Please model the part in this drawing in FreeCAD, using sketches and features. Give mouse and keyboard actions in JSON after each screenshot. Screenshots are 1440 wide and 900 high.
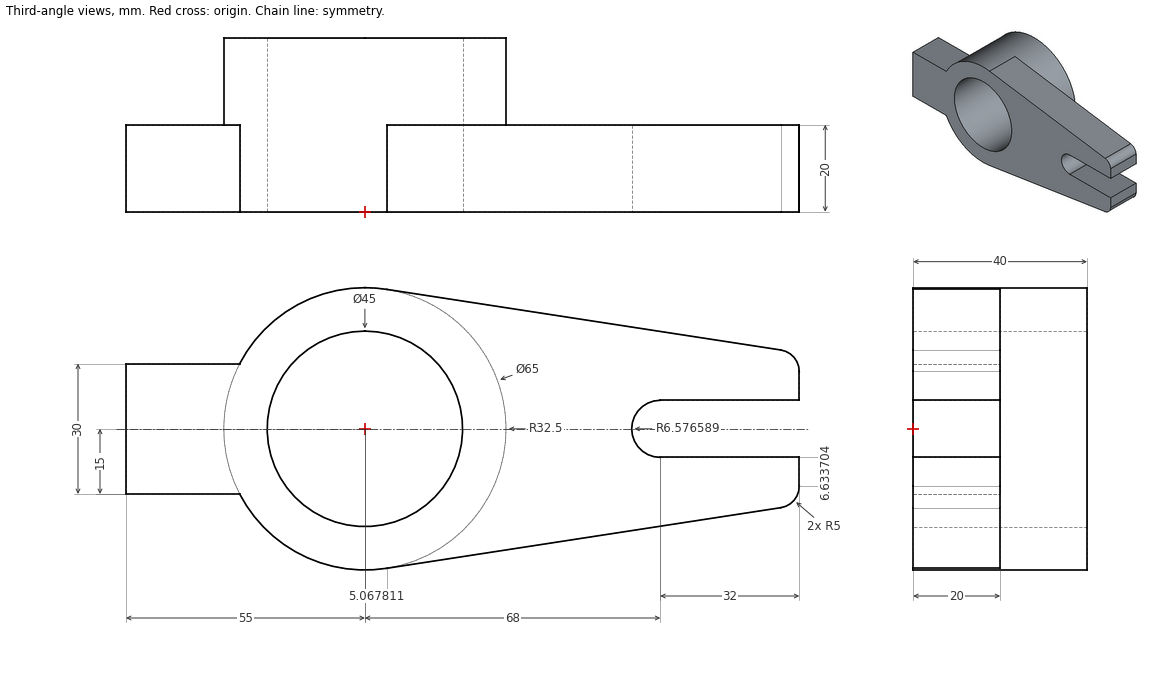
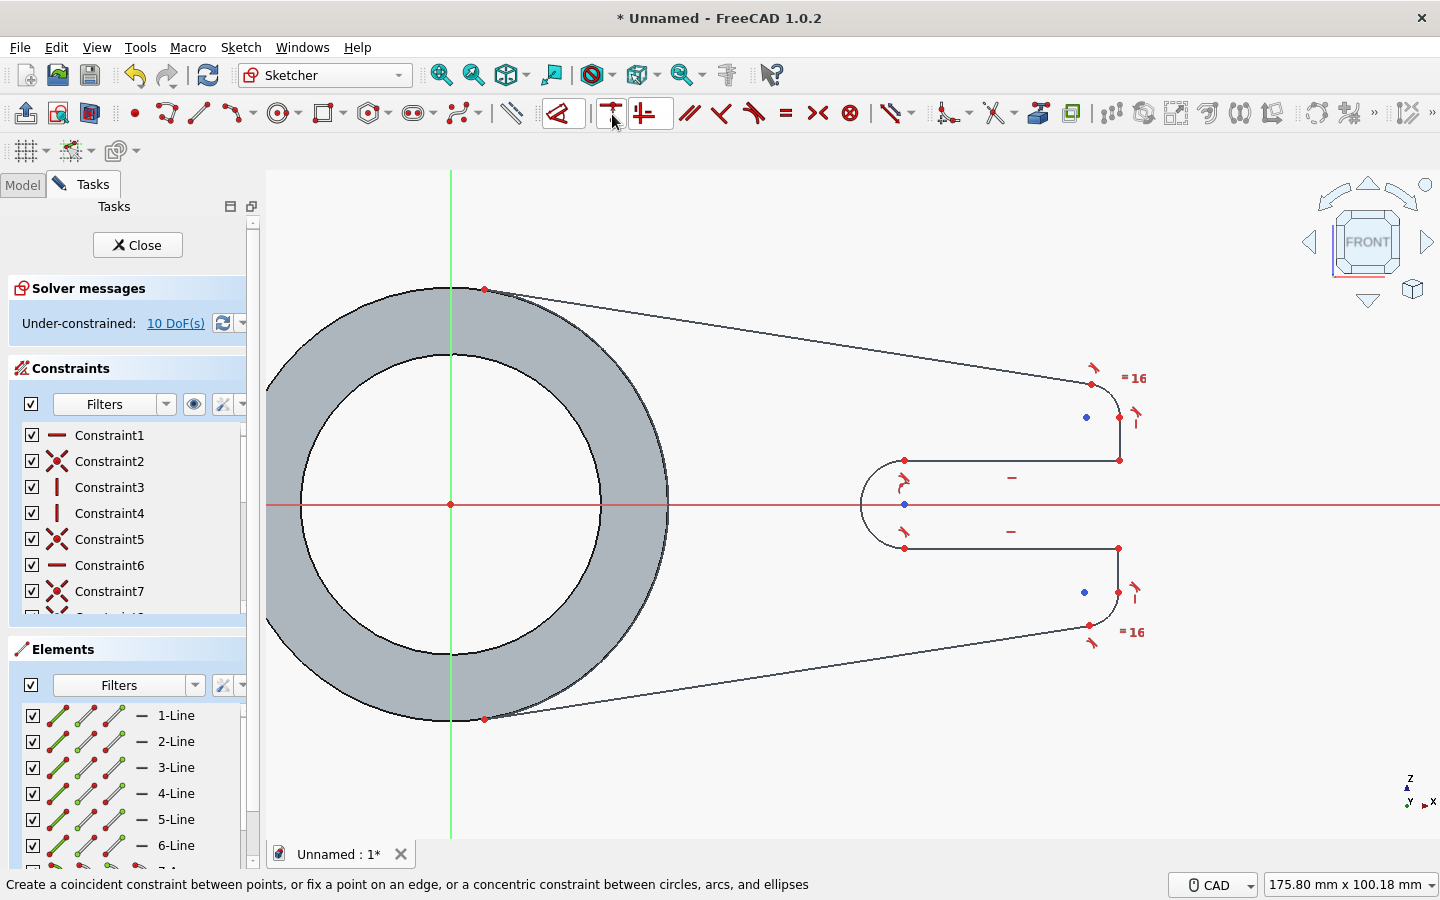
{"action": "left_click", "coordinate": [1085, 593]}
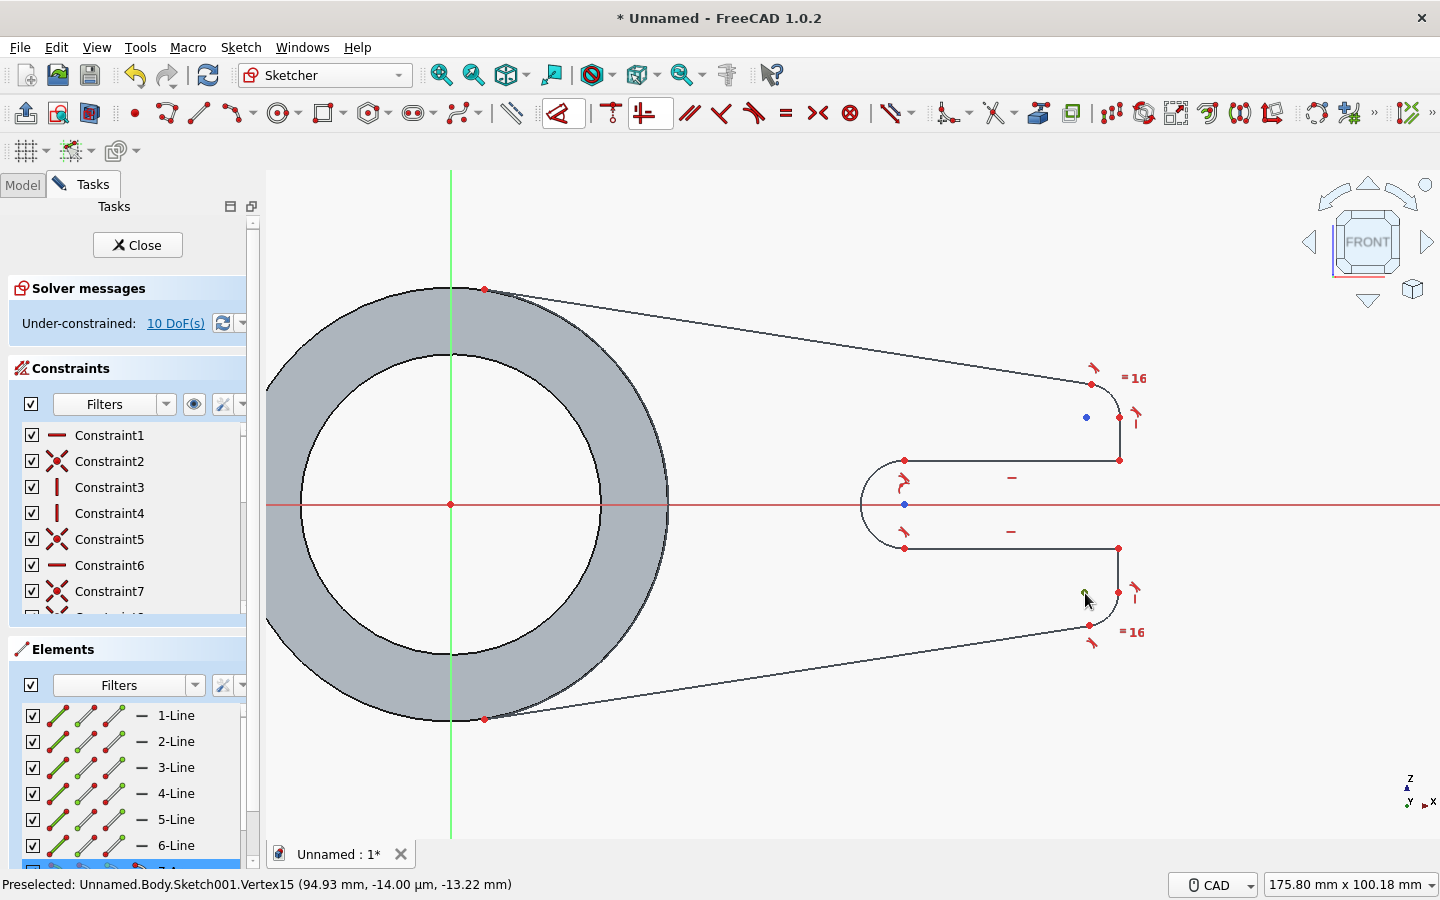
{"action": "left_click", "coordinate": [1086, 418]}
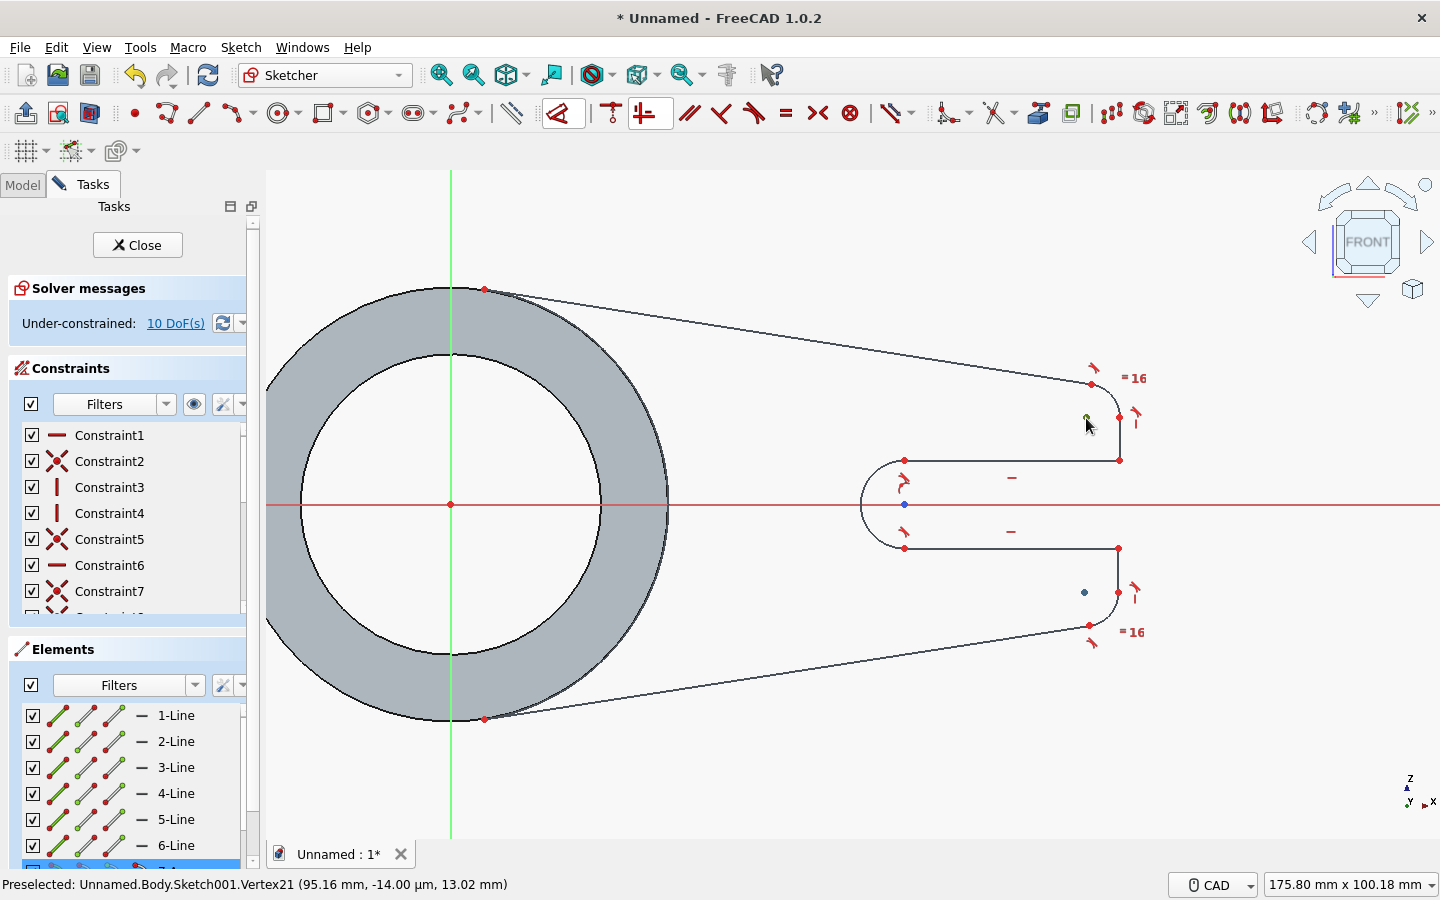
{"action": "left_click", "coordinate": [364, 505]}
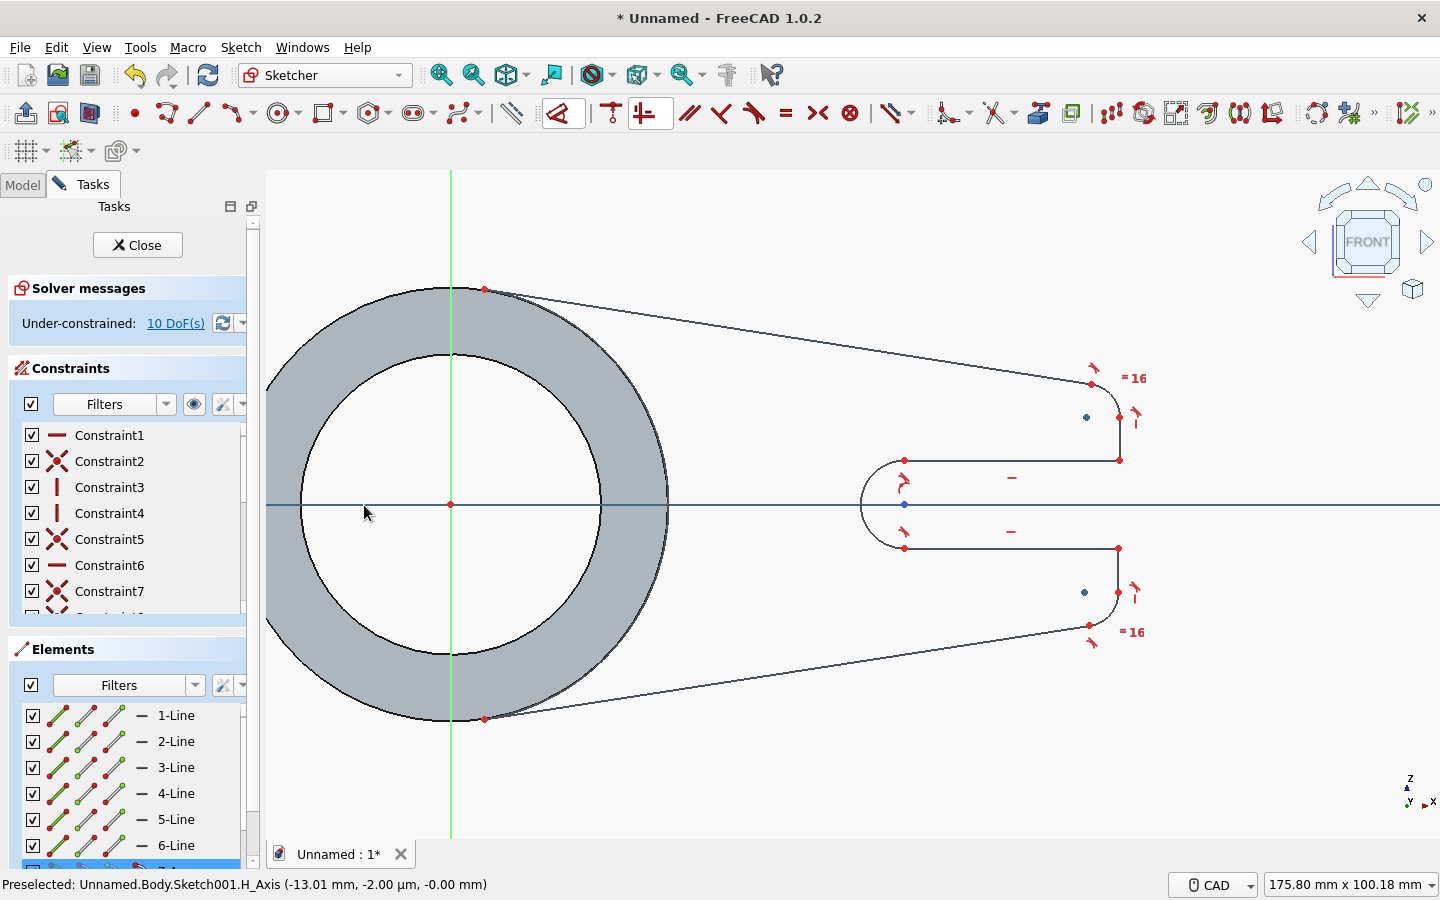
{"action": "left_click", "coordinate": [818, 114]}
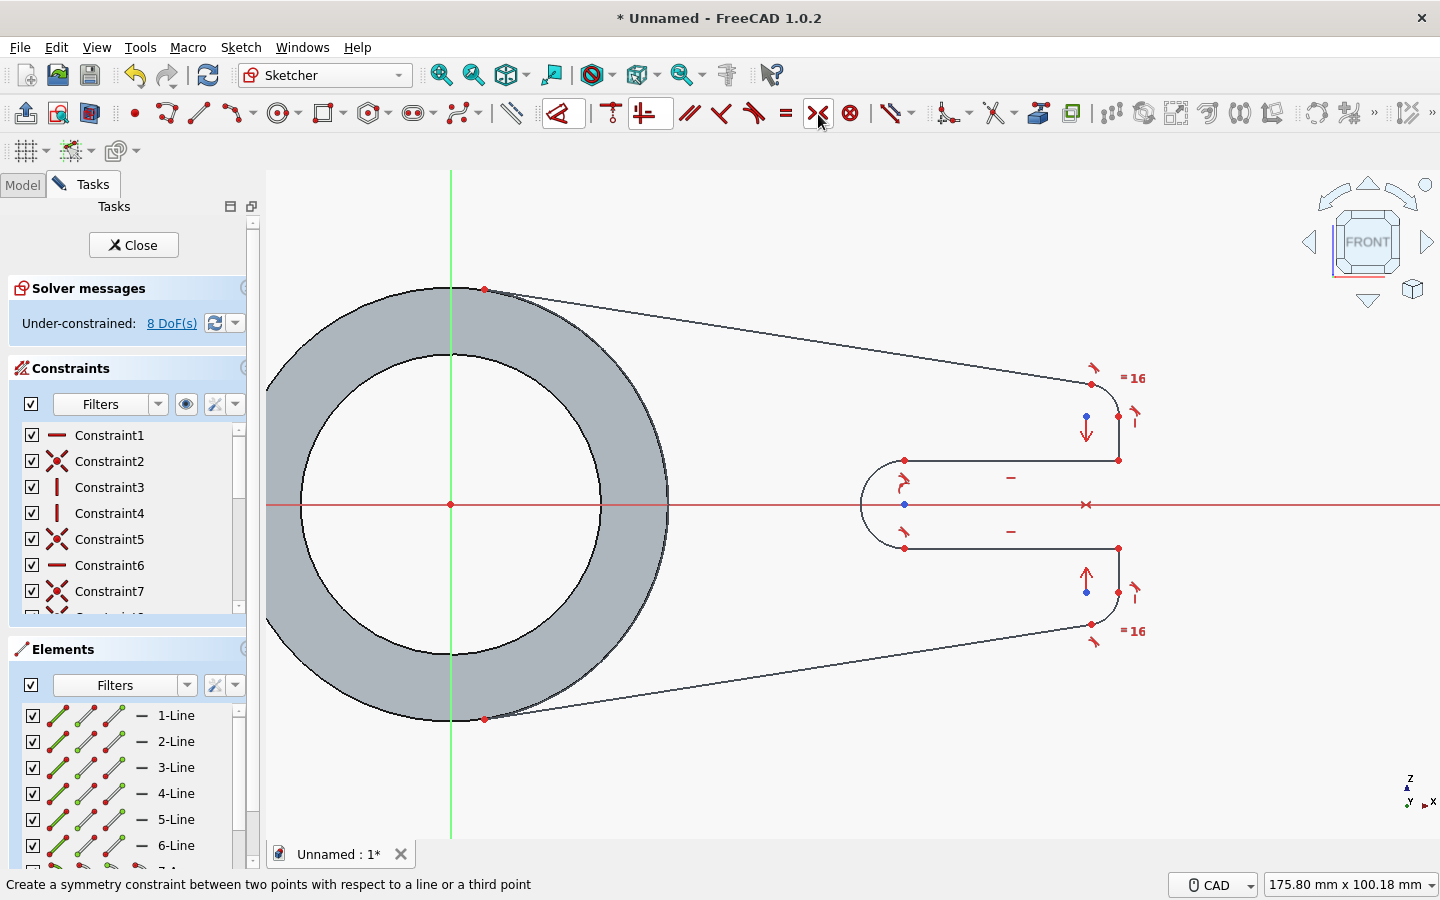
{"action": "key", "text": "d"}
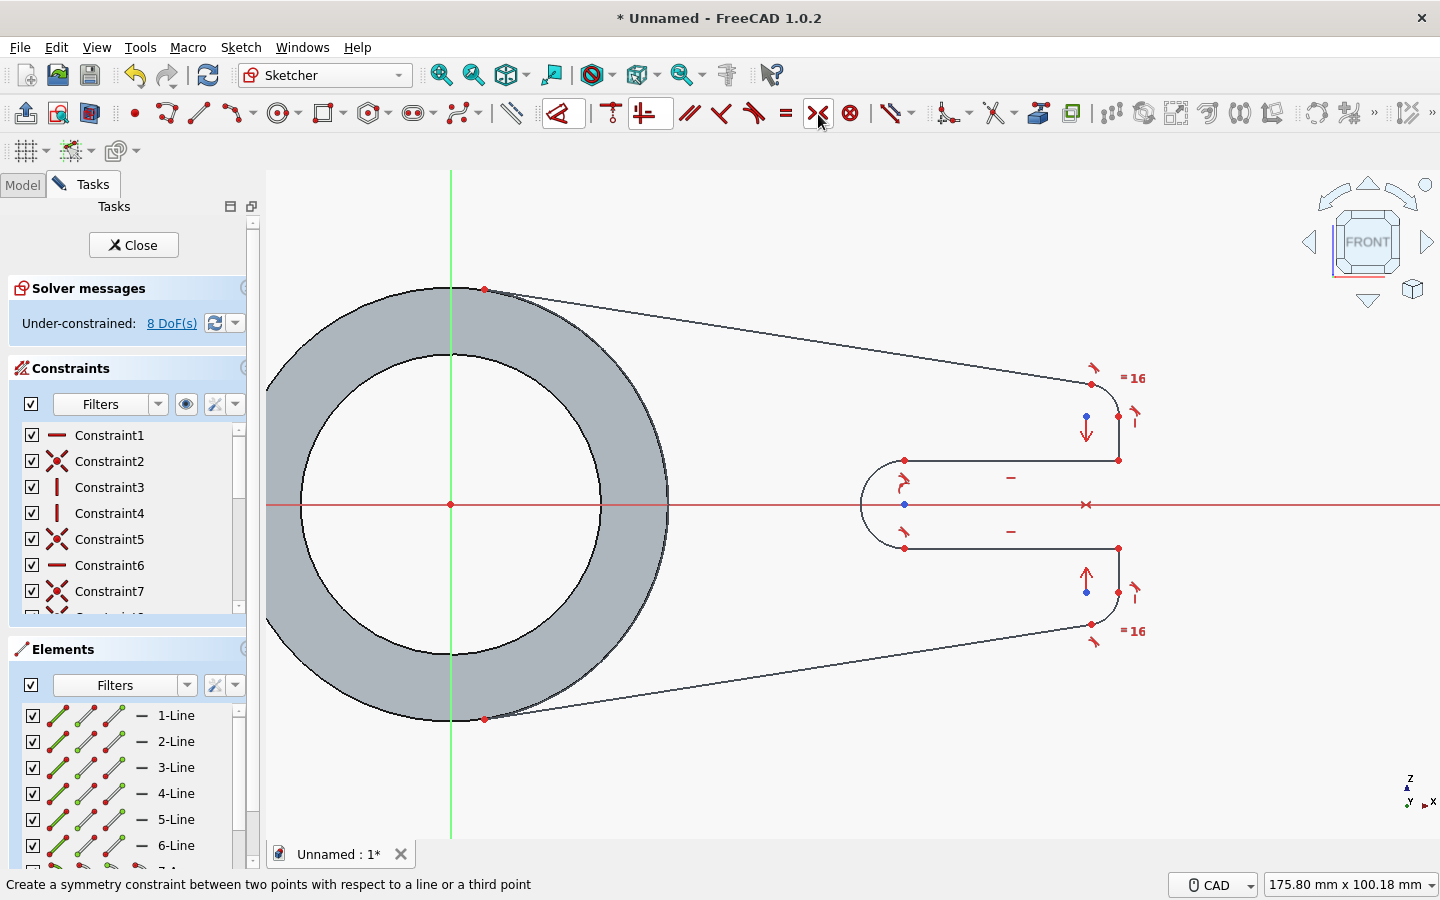
{"action": "left_click", "coordinate": [1104, 620]}
{"action": "left_click", "coordinate": [1121, 647]}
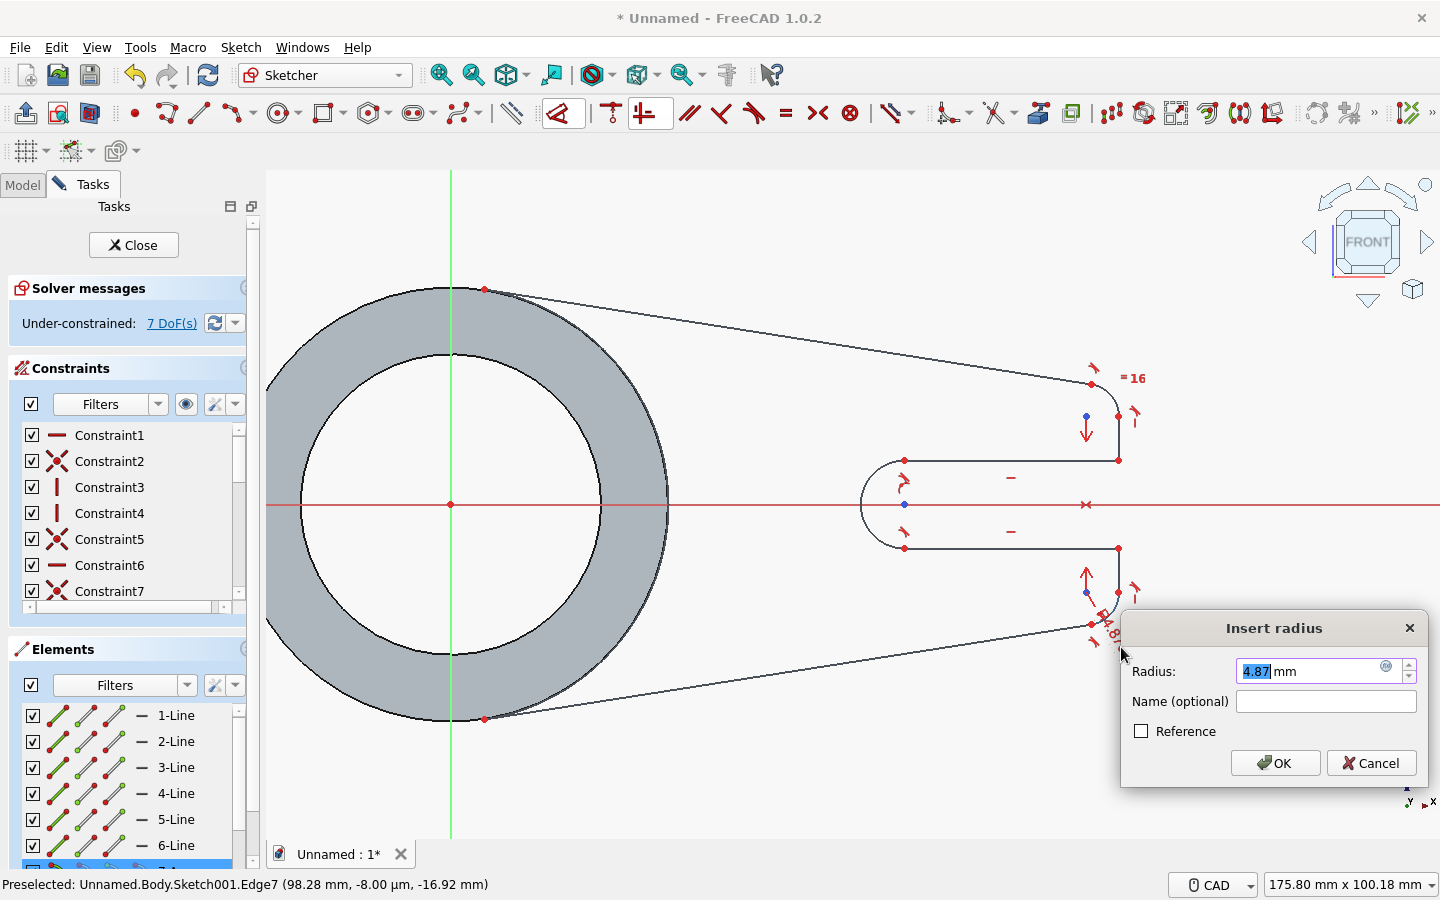
{"action": "type", "text": "5"}
{"action": "key", "text": "Return"}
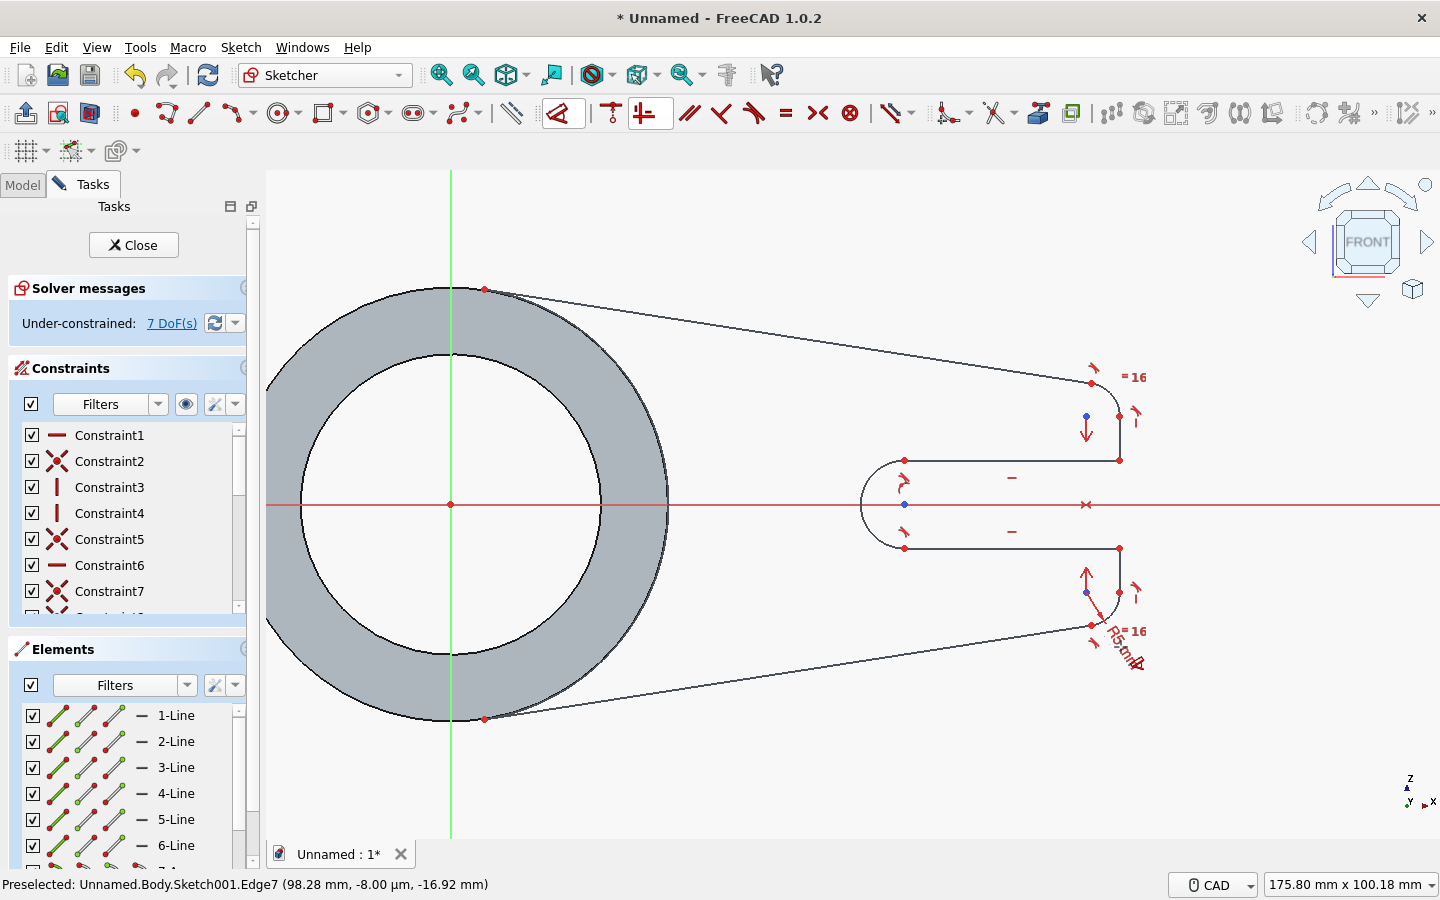
{"action": "left_click", "coordinate": [635, 621]}
{"action": "left_click", "coordinate": [662, 638]}